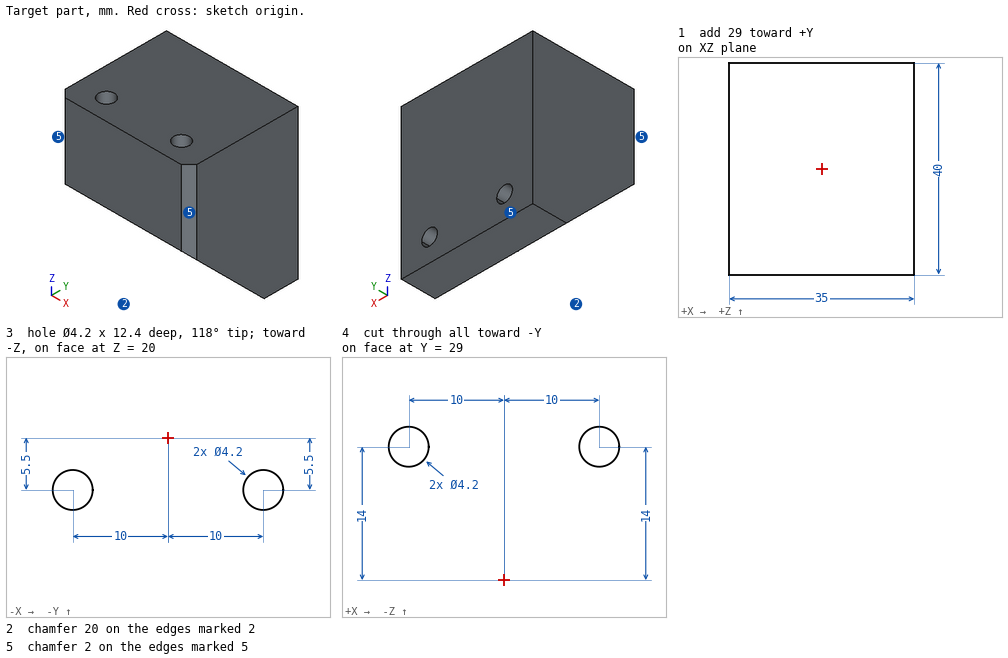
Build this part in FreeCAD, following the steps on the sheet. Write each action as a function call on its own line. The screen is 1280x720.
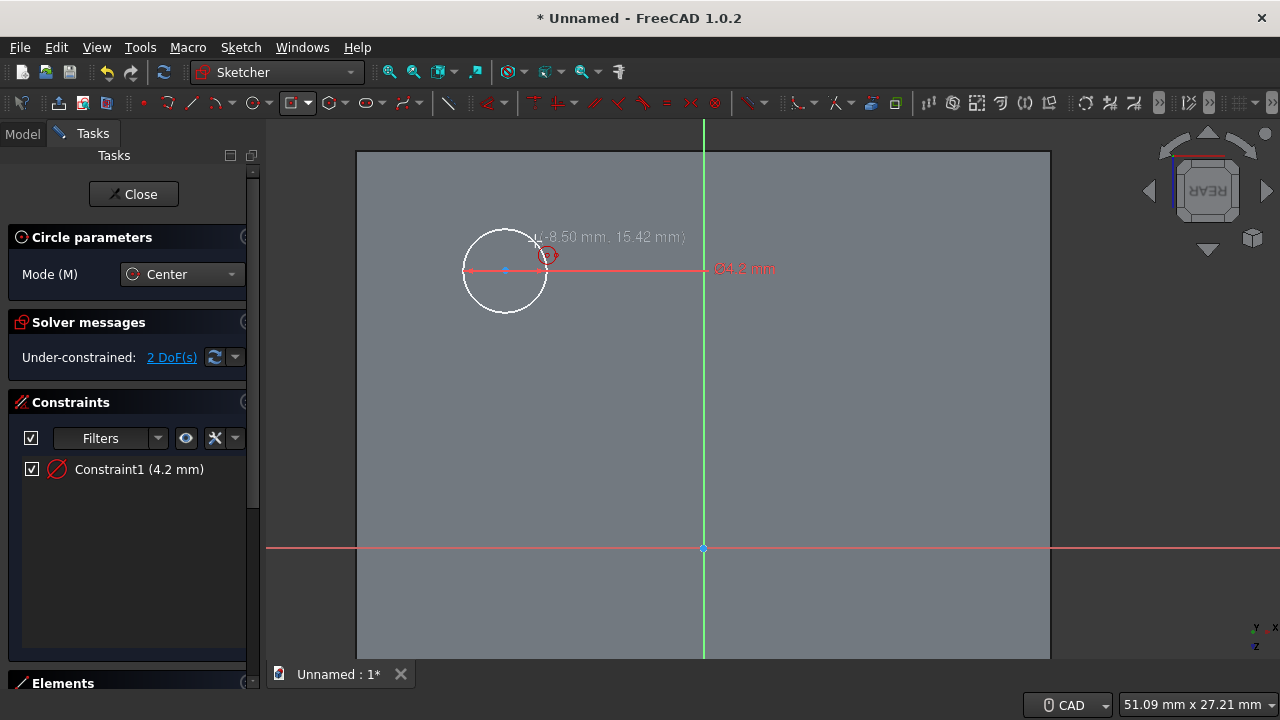
click(902, 270)
move(932, 241)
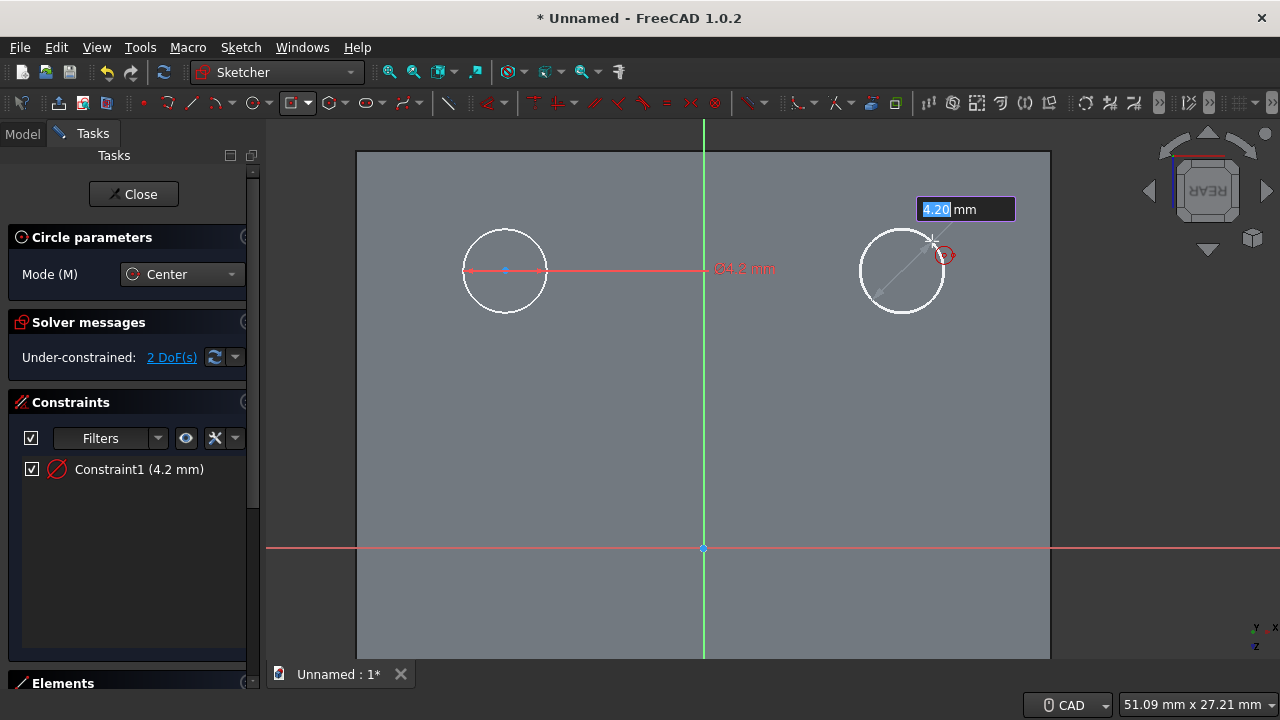
text(4.2)
key(Return)
key(Escape)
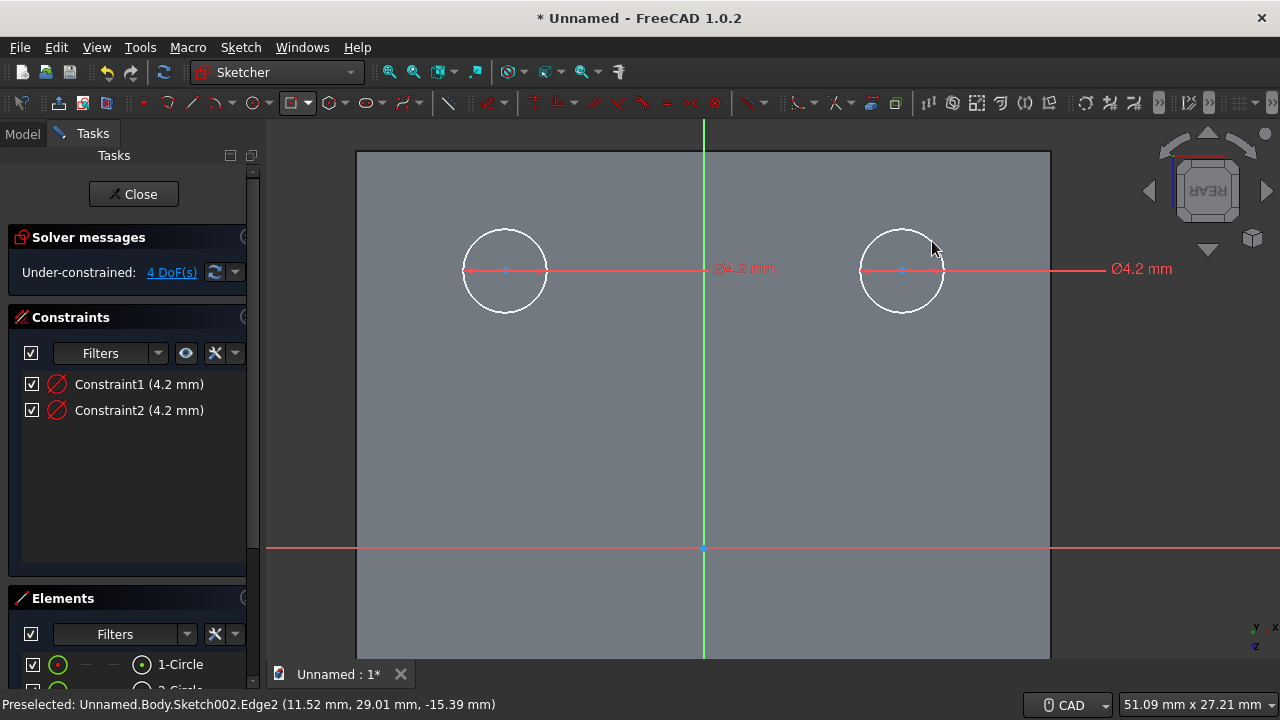
click(488, 104)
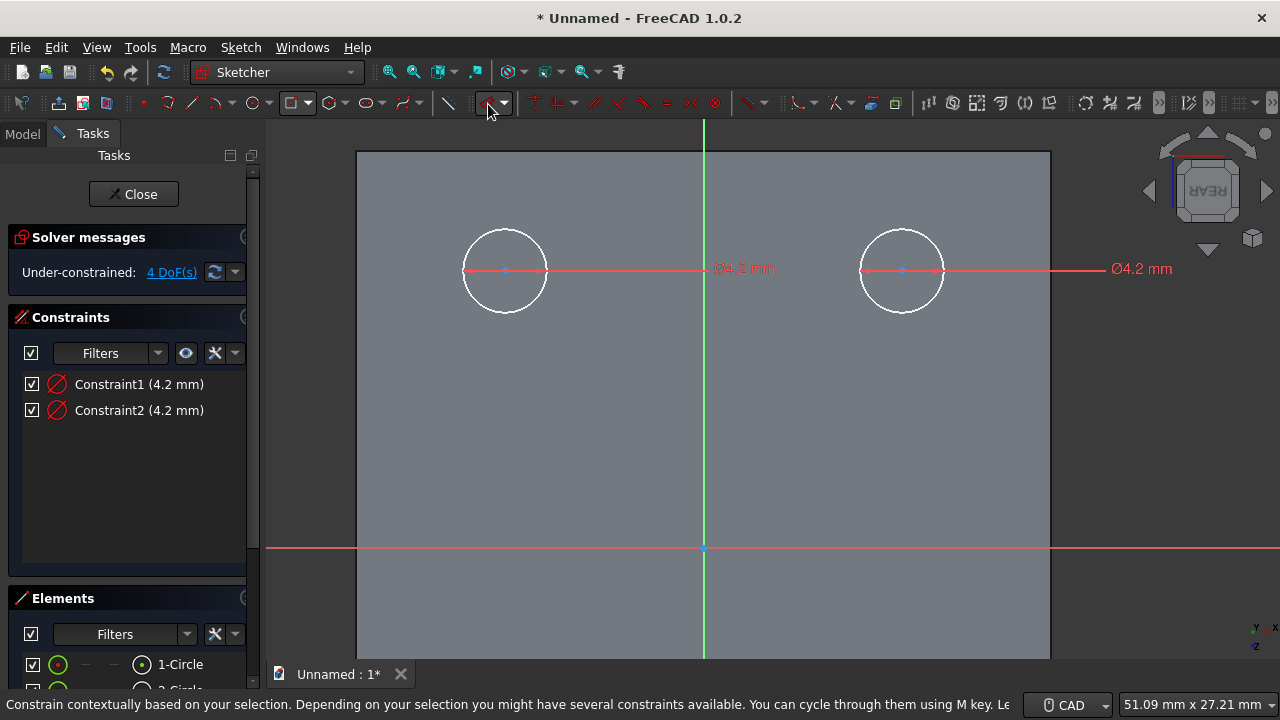
click(505, 271)
click(604, 582)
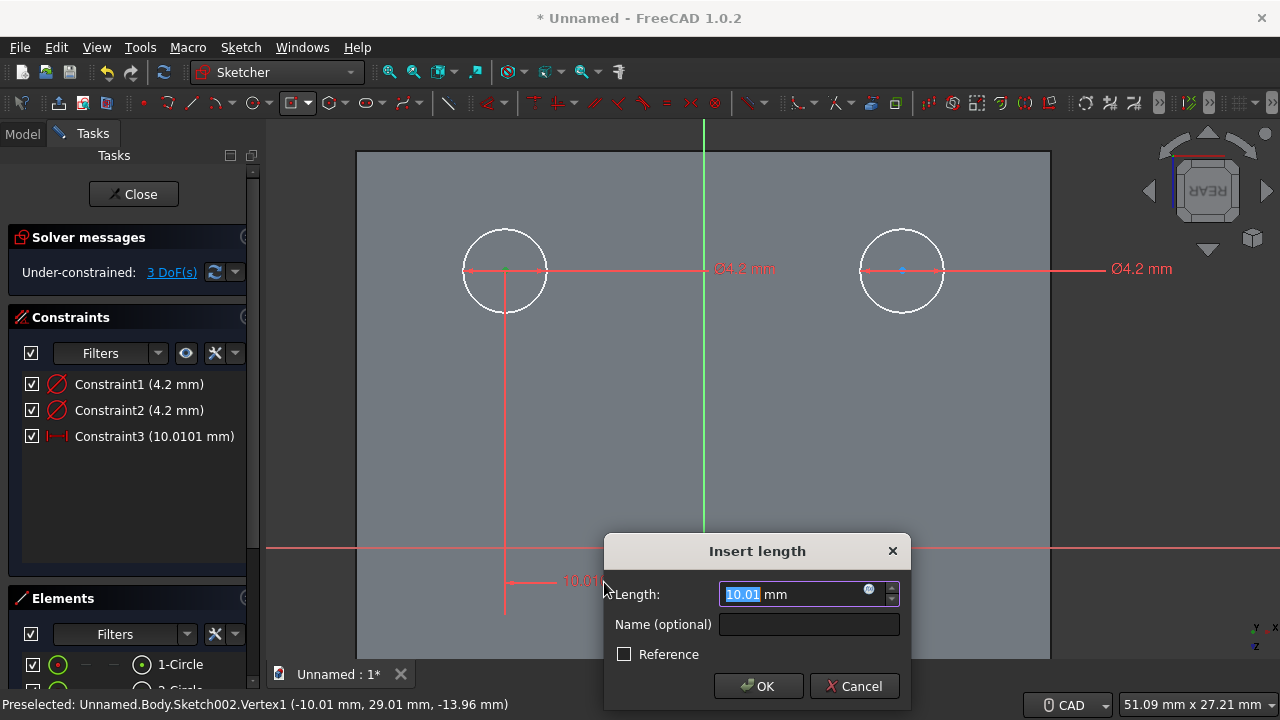
text(10)
key(Return)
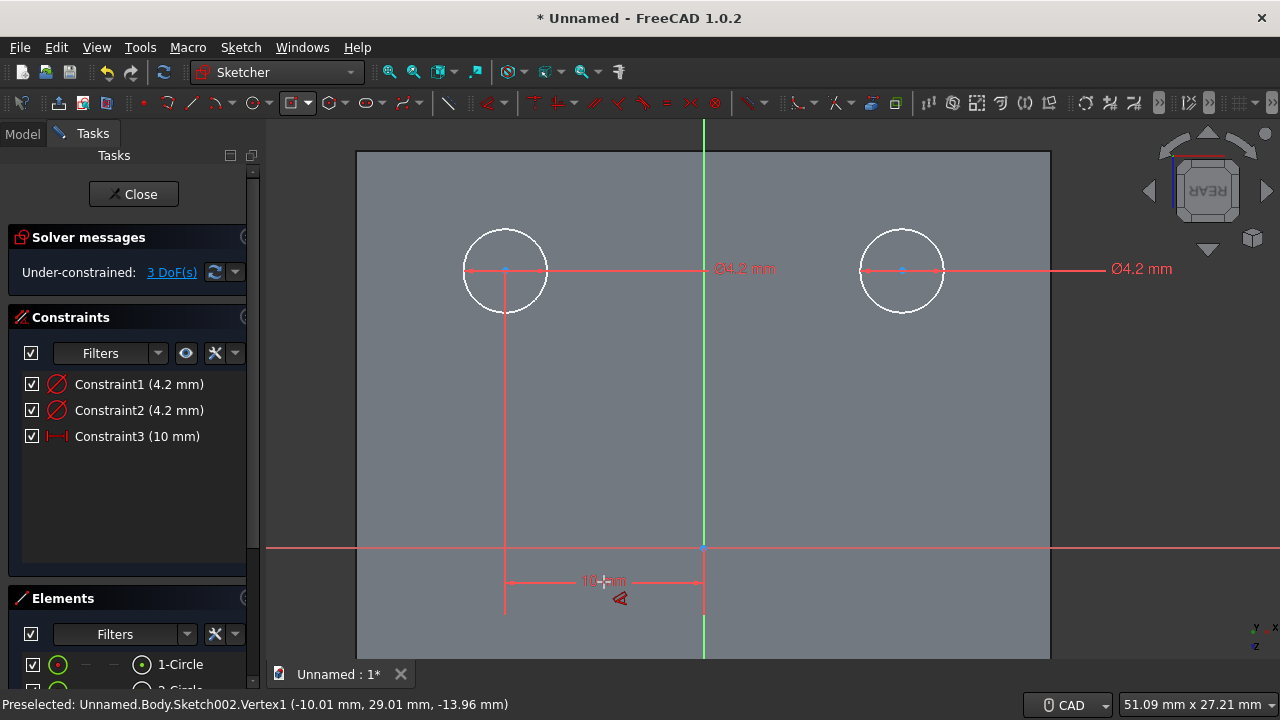
click(505, 271)
click(471, 410)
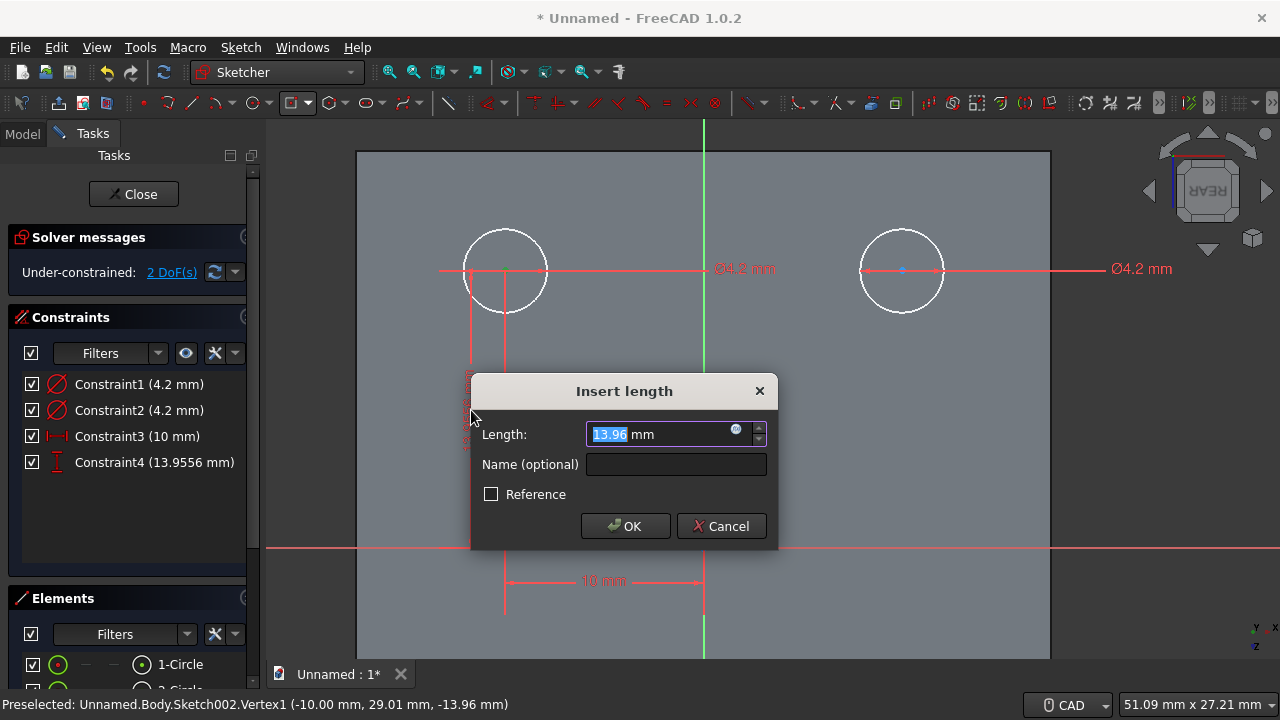
text(14)
key(Return)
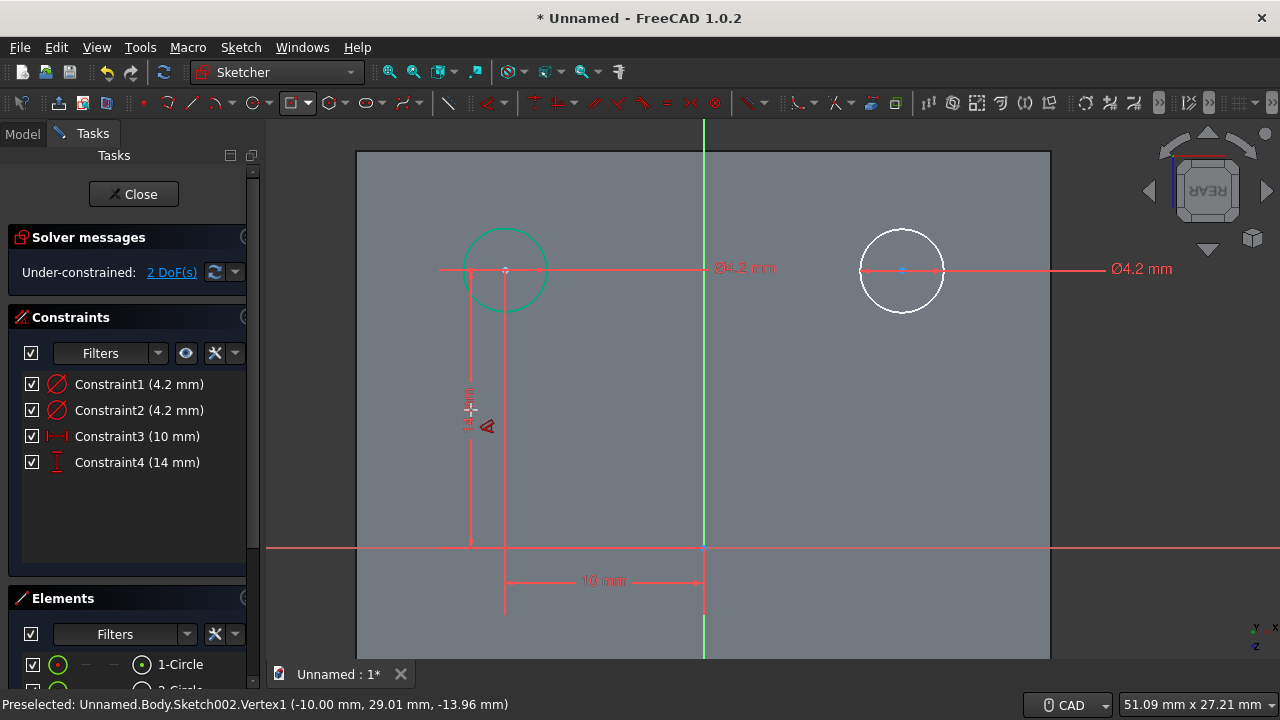
click(902, 271)
click(803, 582)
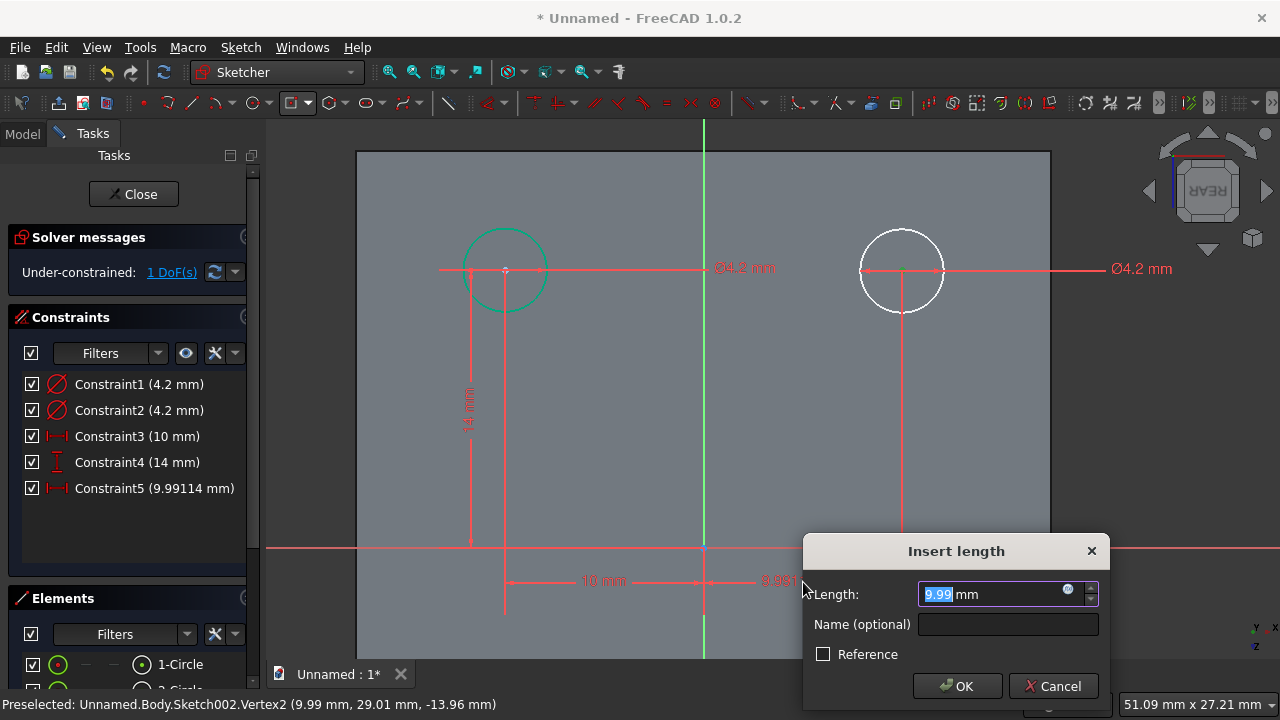
text(10)
key(Return)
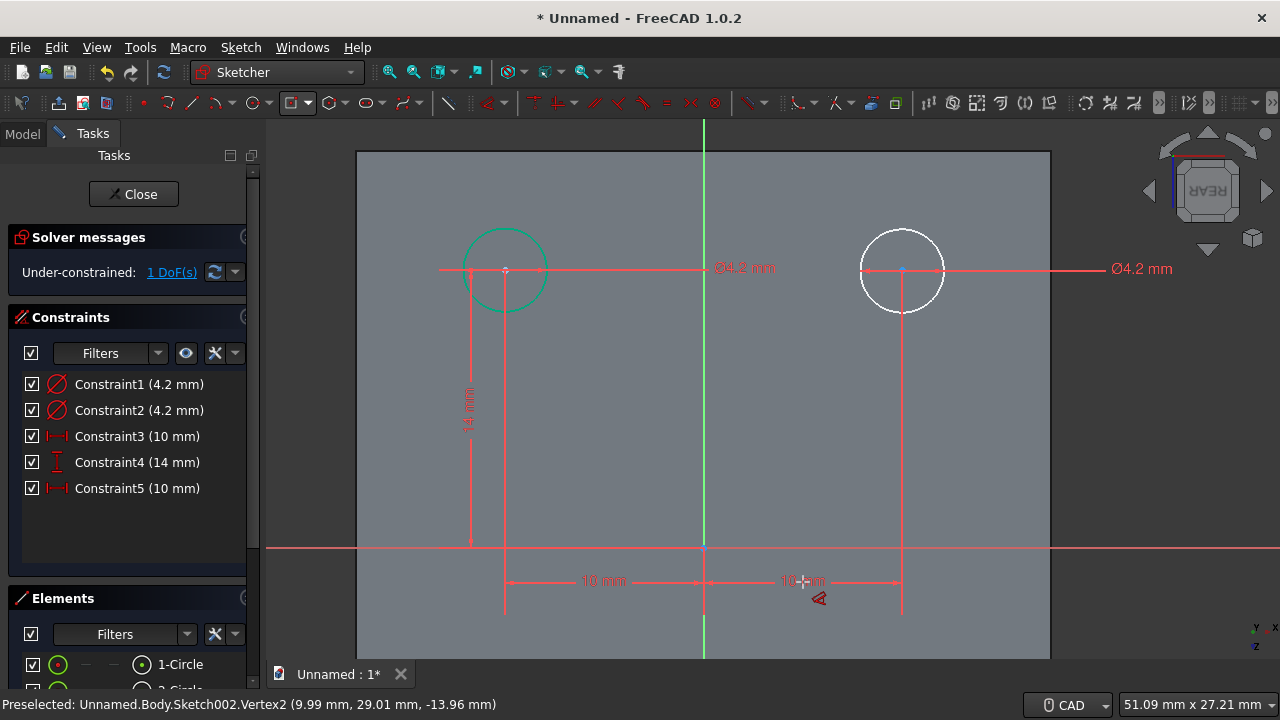
click(902, 271)
click(936, 410)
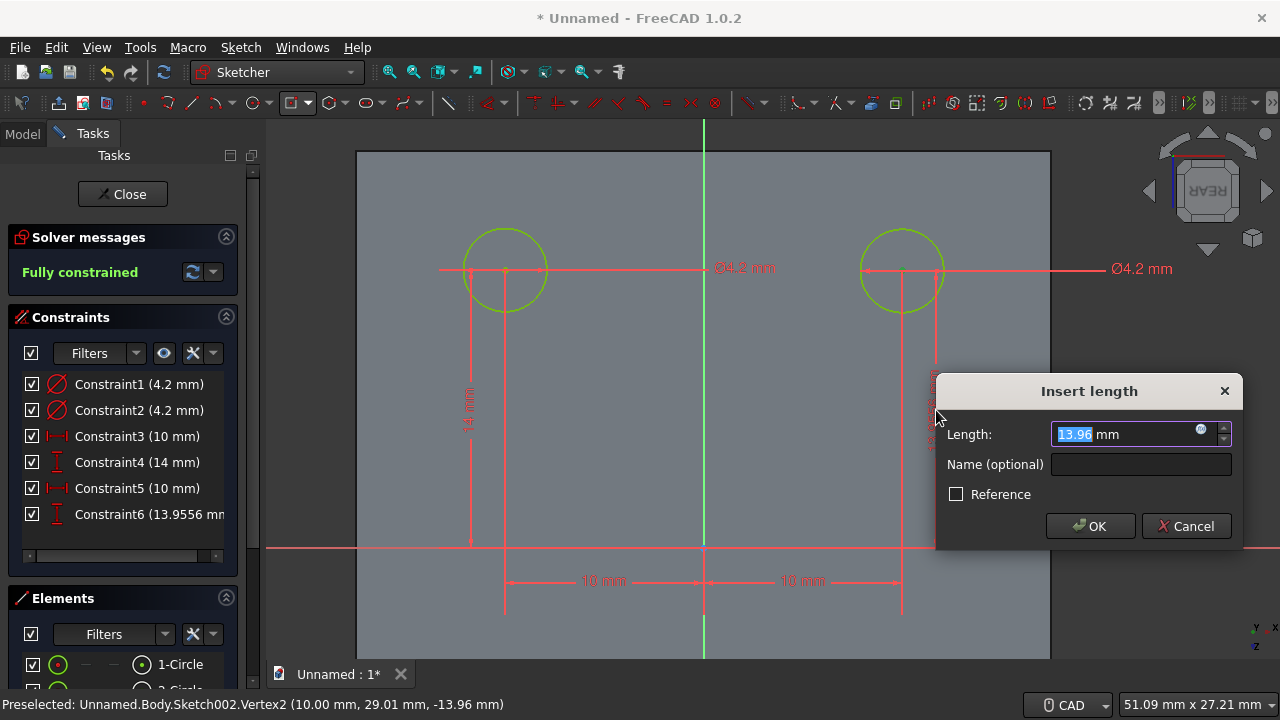
text(14)
key(Return)
key(Escape)